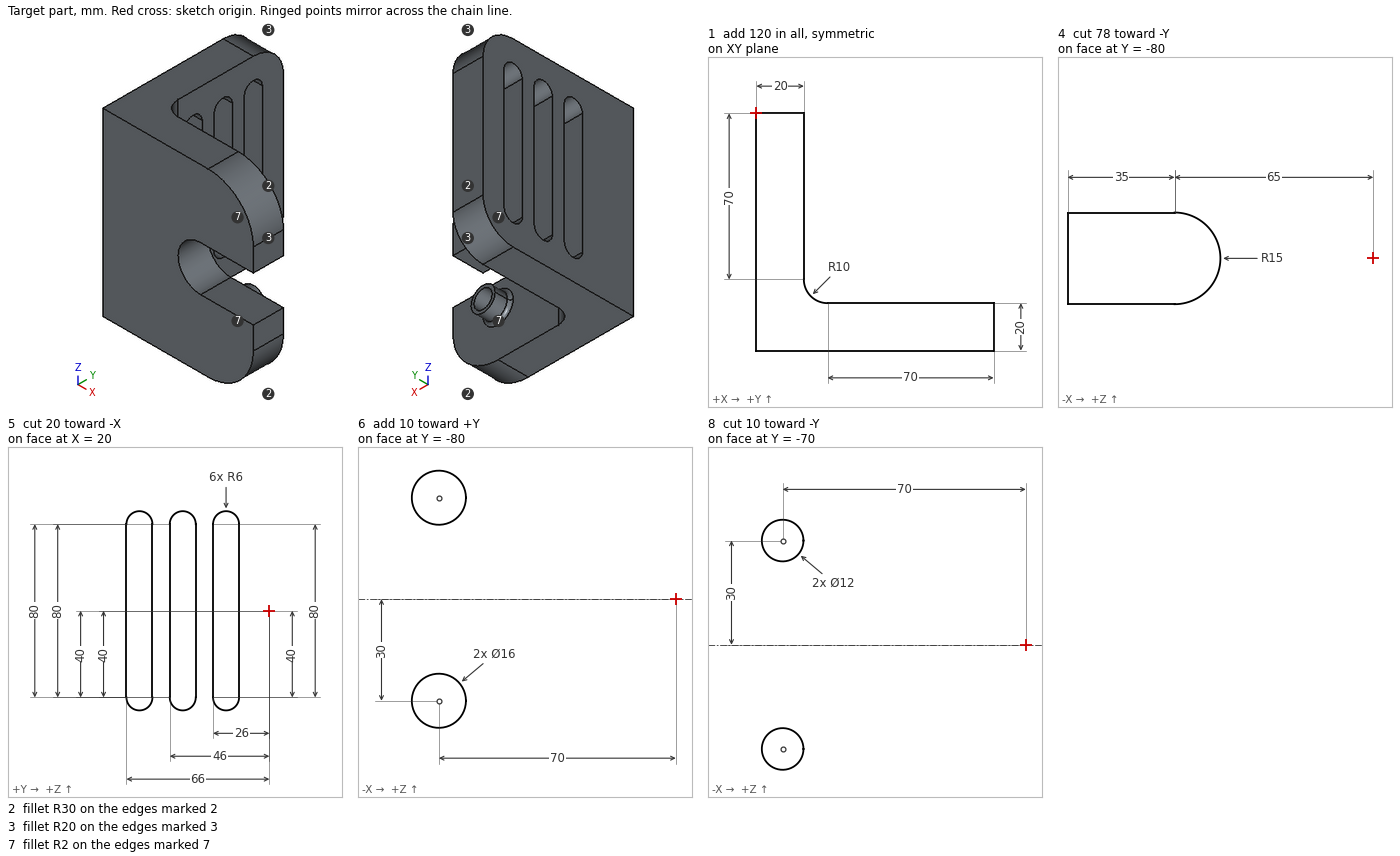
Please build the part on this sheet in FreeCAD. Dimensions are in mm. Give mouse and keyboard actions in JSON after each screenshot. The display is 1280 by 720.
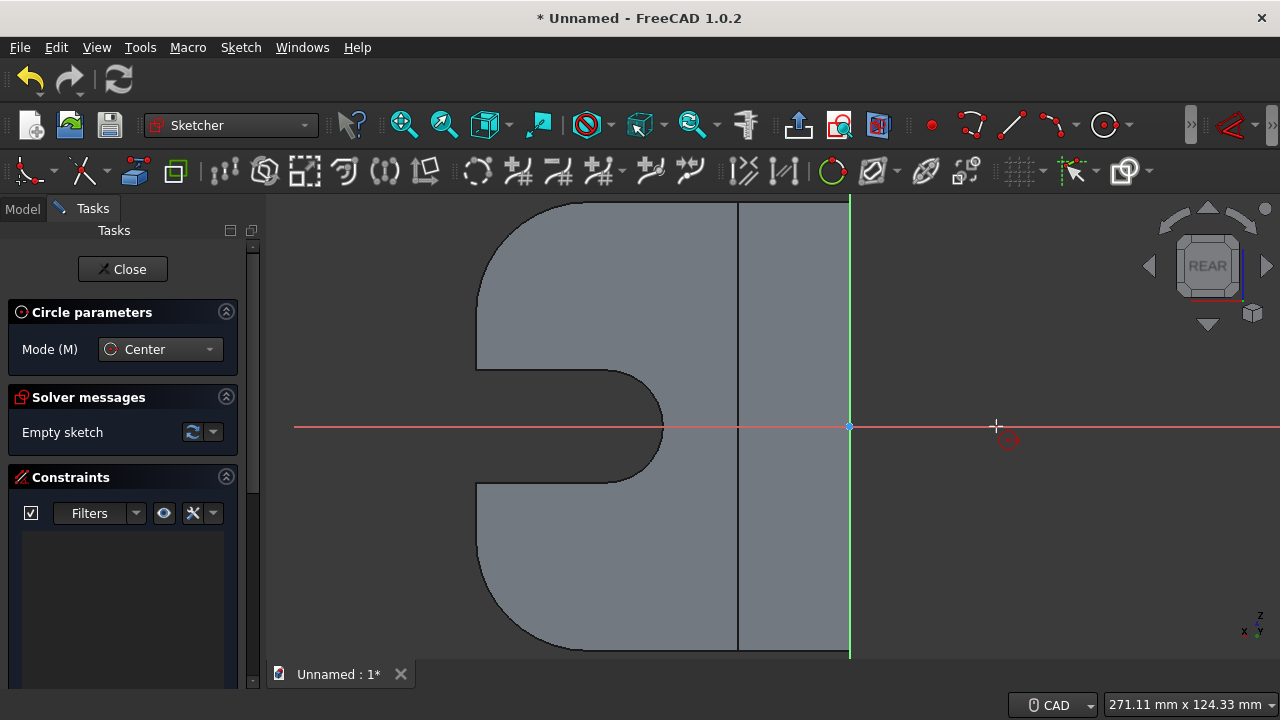
{"action": "left_click", "coordinate": [588, 539]}
{"action": "left_click", "coordinate": [609, 518]}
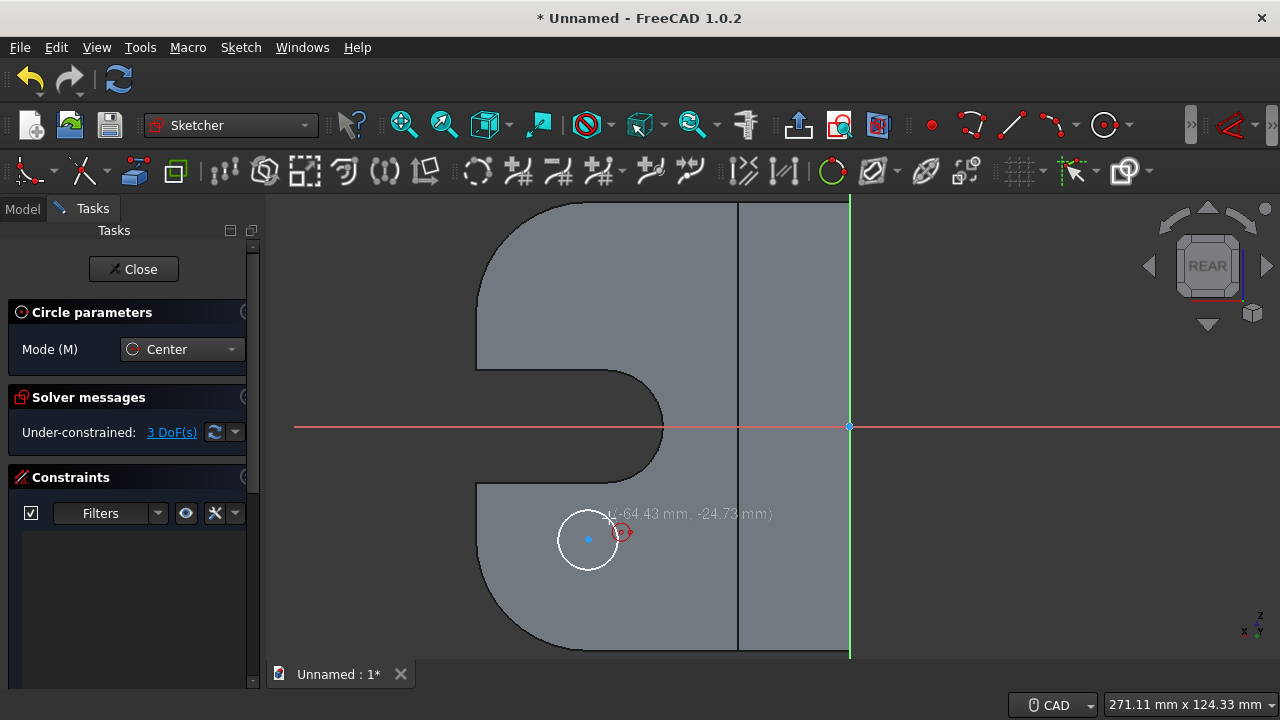
{"action": "left_click", "coordinate": [588, 314]}
{"action": "left_click", "coordinate": [609, 293]}
{"action": "key", "text": "Escape"}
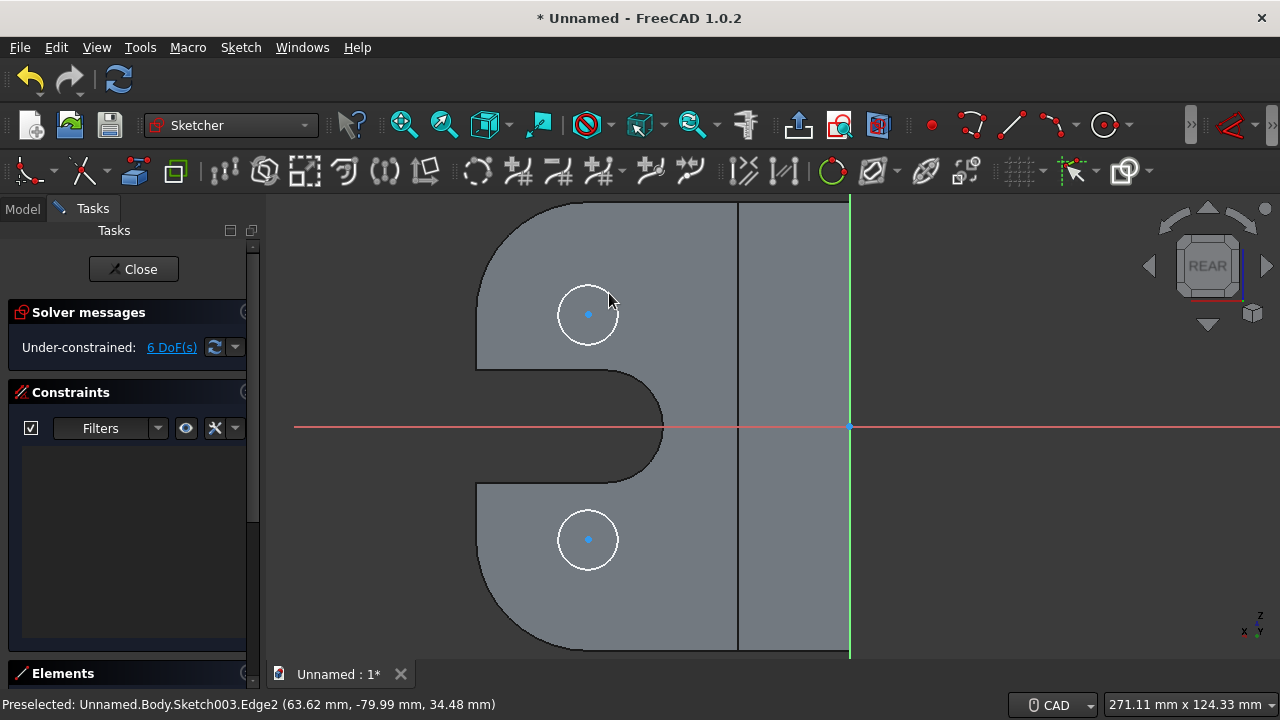
{"action": "left_click", "coordinate": [609, 519]}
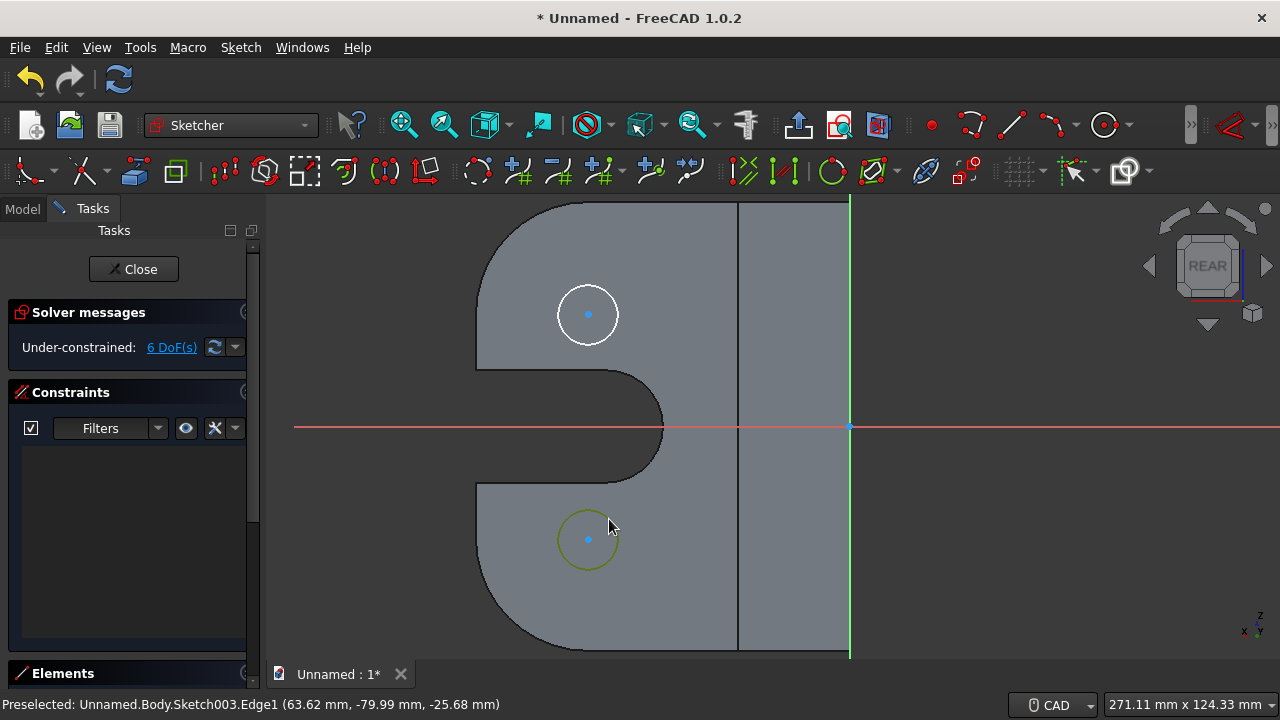
{"action": "left_click", "coordinate": [609, 294]}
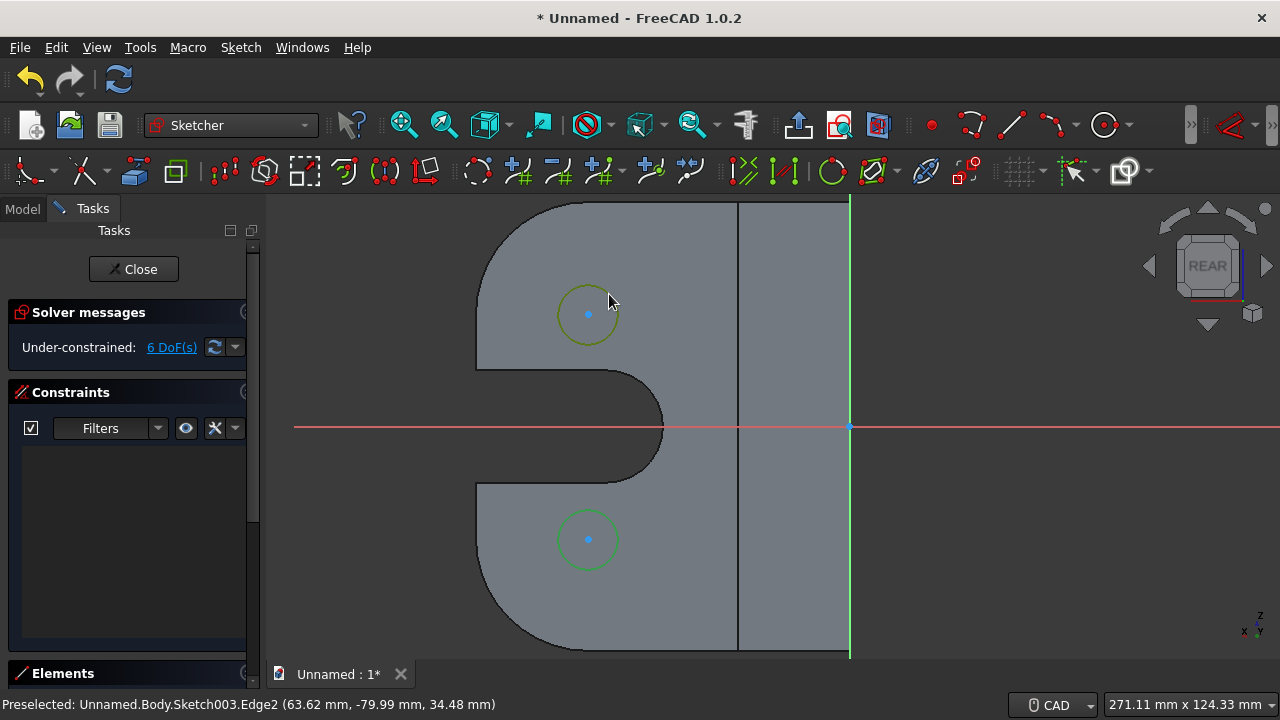
{"action": "key", "text": "e"}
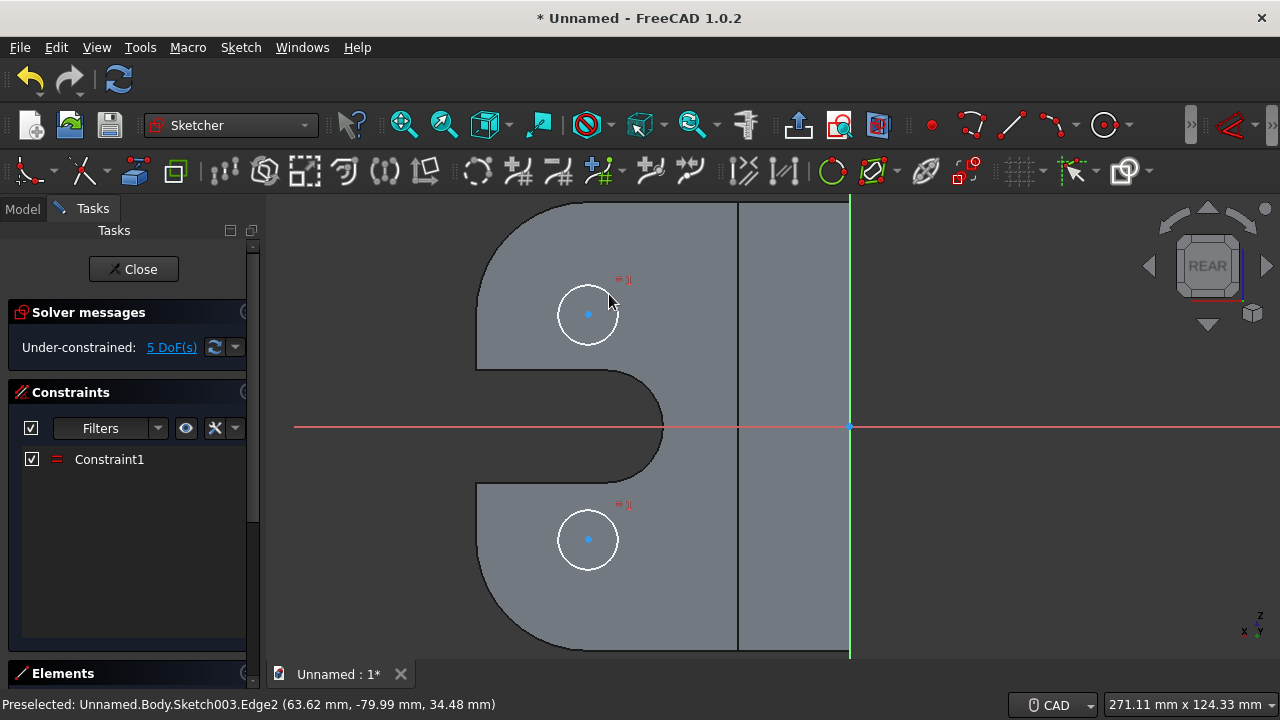
{"action": "left_click", "coordinate": [588, 540]}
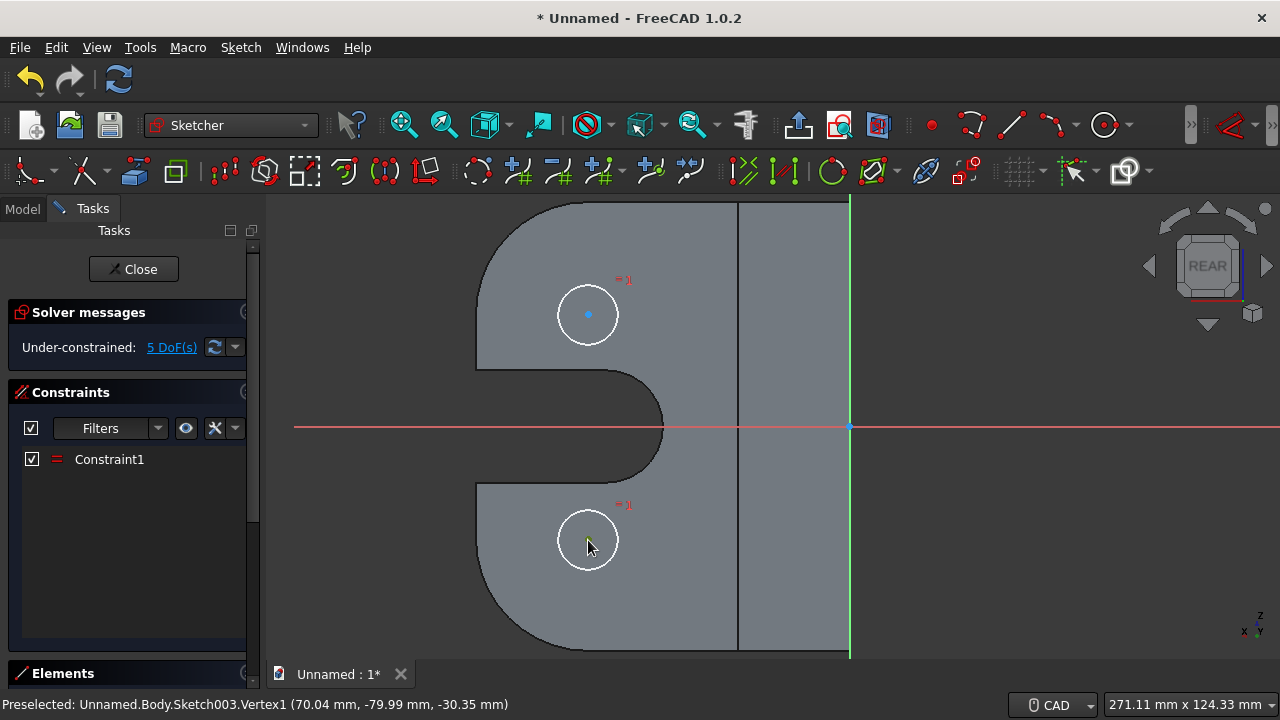
{"action": "left_click", "coordinate": [588, 315]}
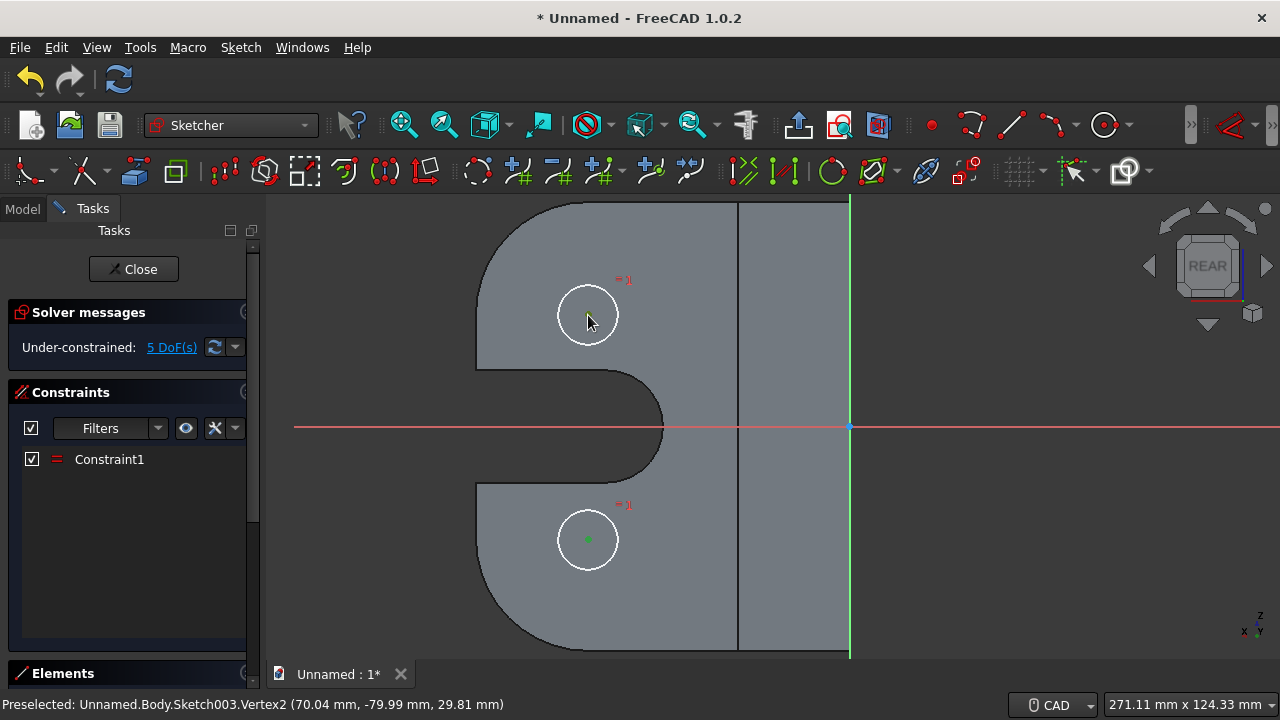
{"action": "left_click", "coordinate": [353, 426]}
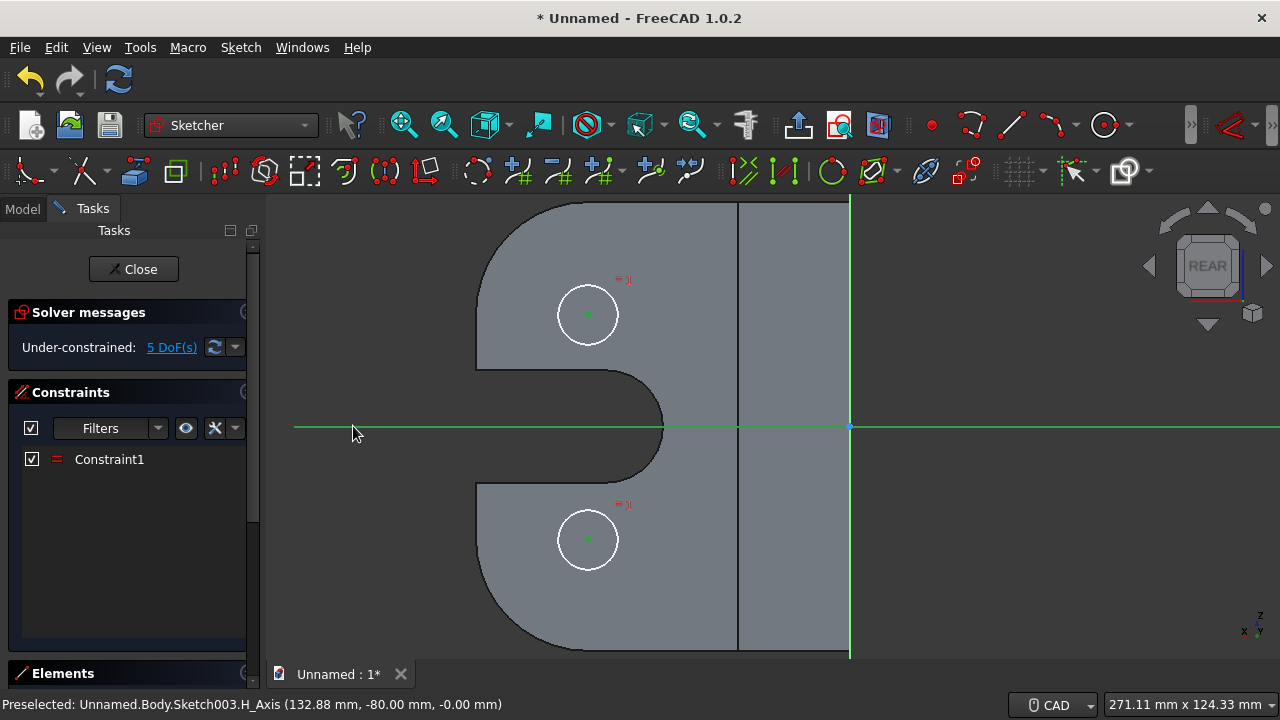
{"action": "key", "text": "s"}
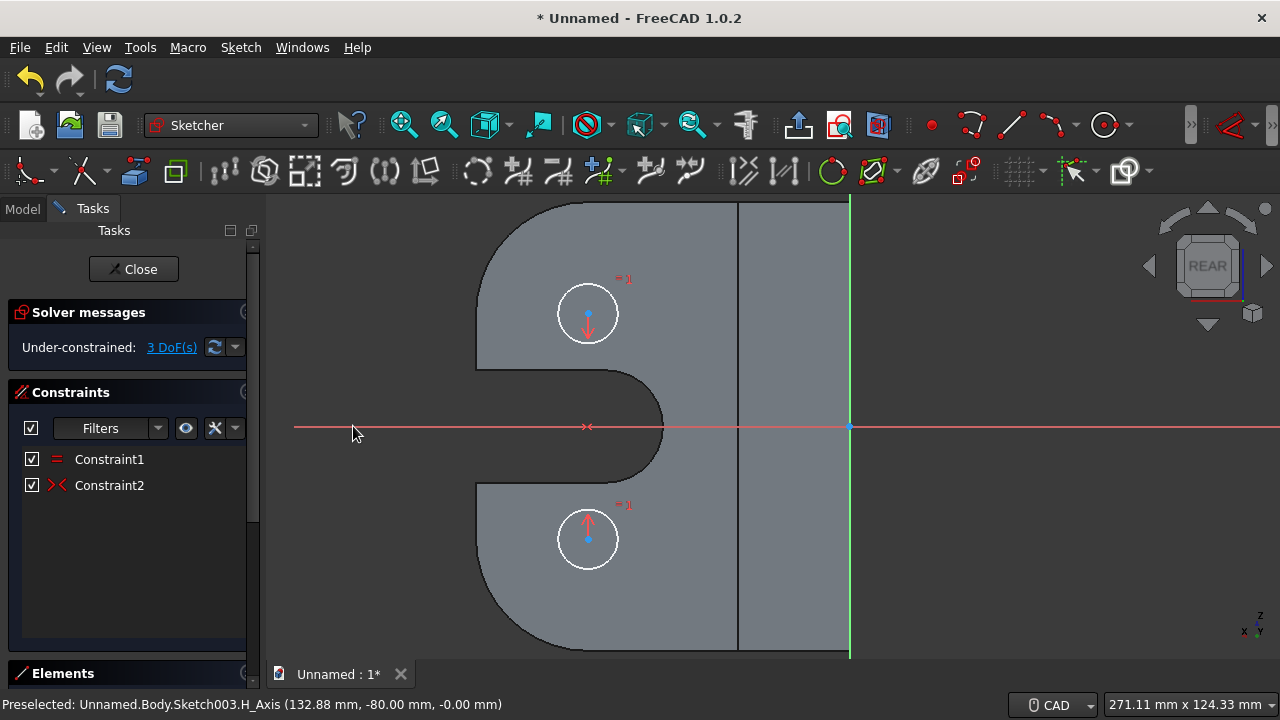
{"action": "left_click", "coordinate": [1230, 126]}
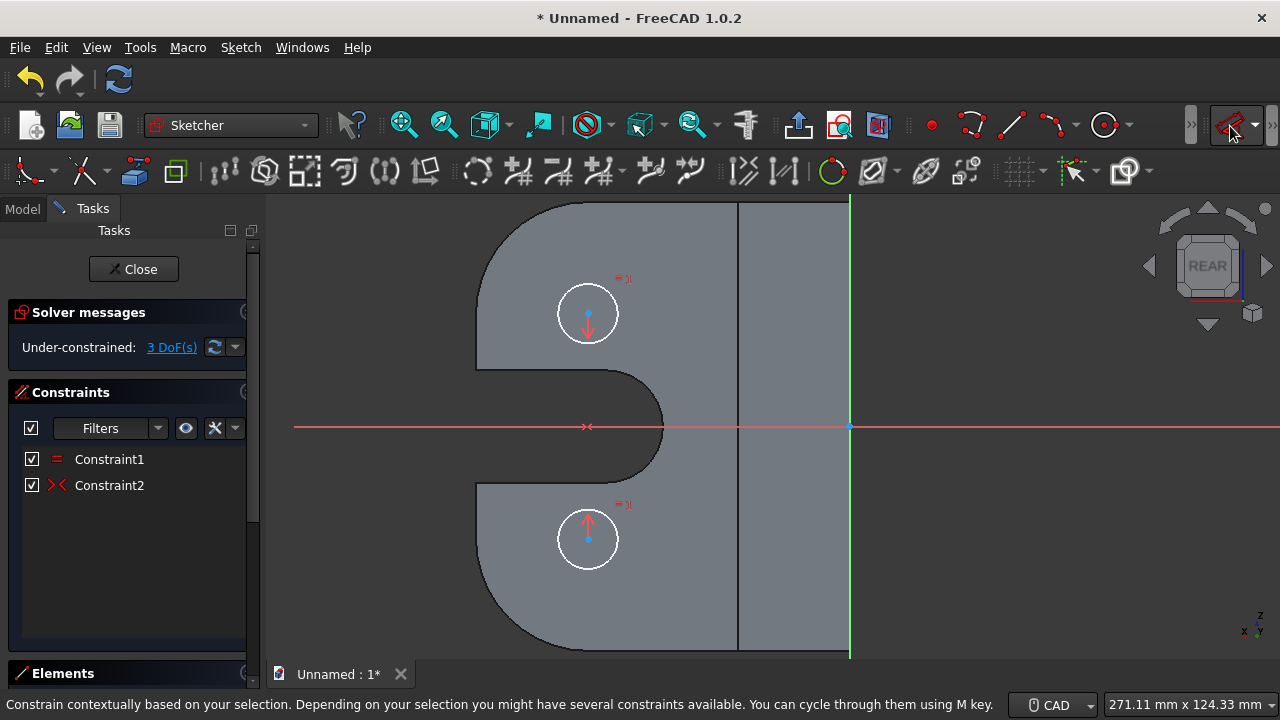
{"action": "left_click", "coordinate": [609, 518]}
{"action": "left_click", "coordinate": [631, 495]}